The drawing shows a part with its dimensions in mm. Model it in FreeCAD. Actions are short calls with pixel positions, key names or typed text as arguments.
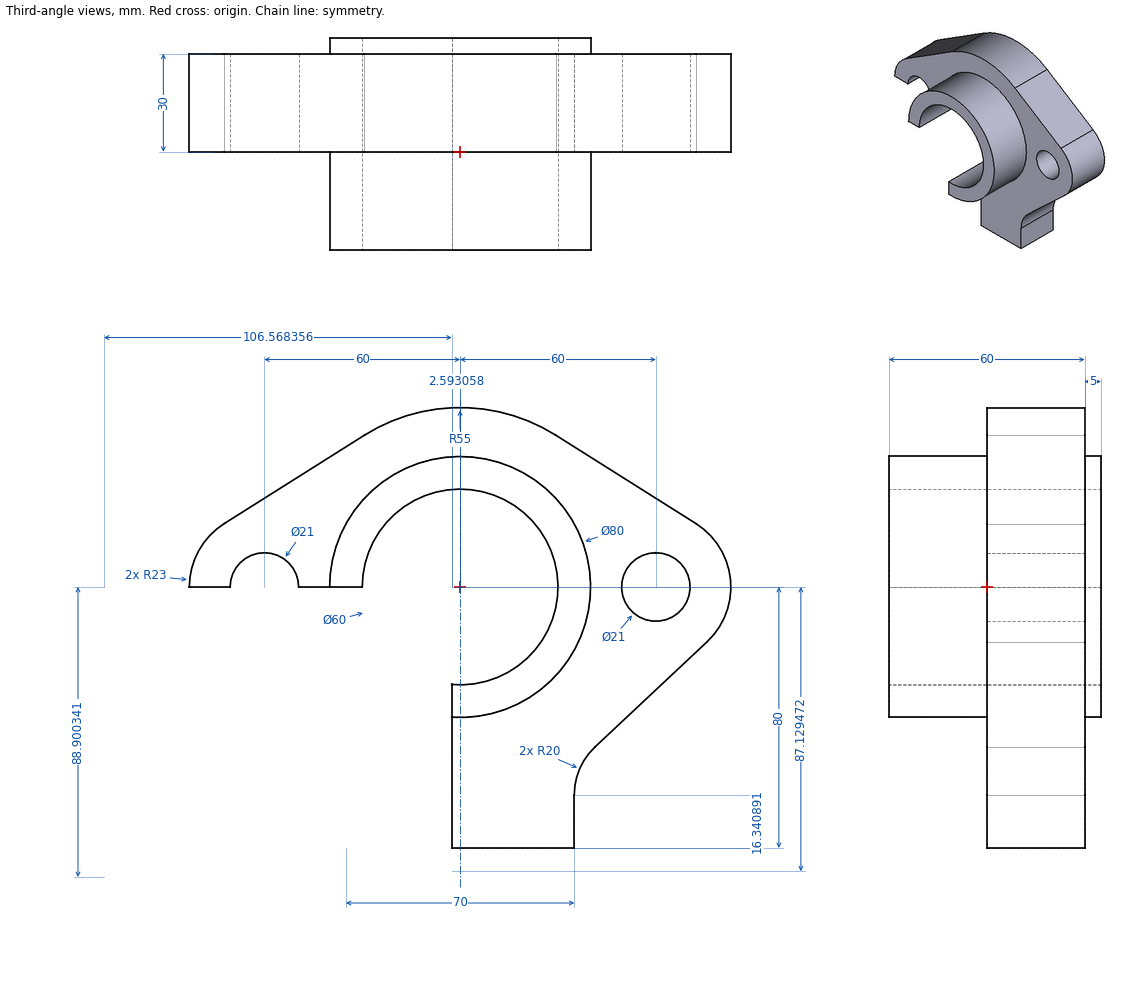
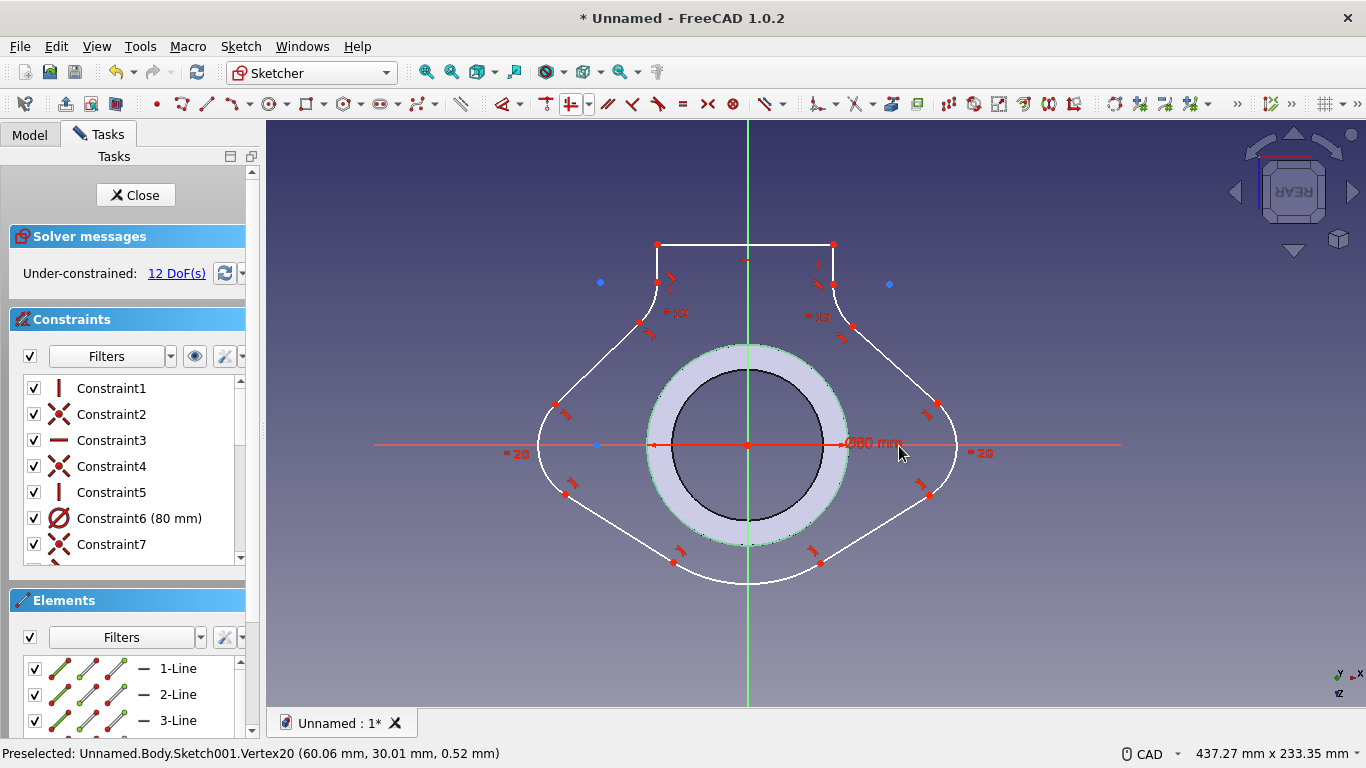
click(424, 445)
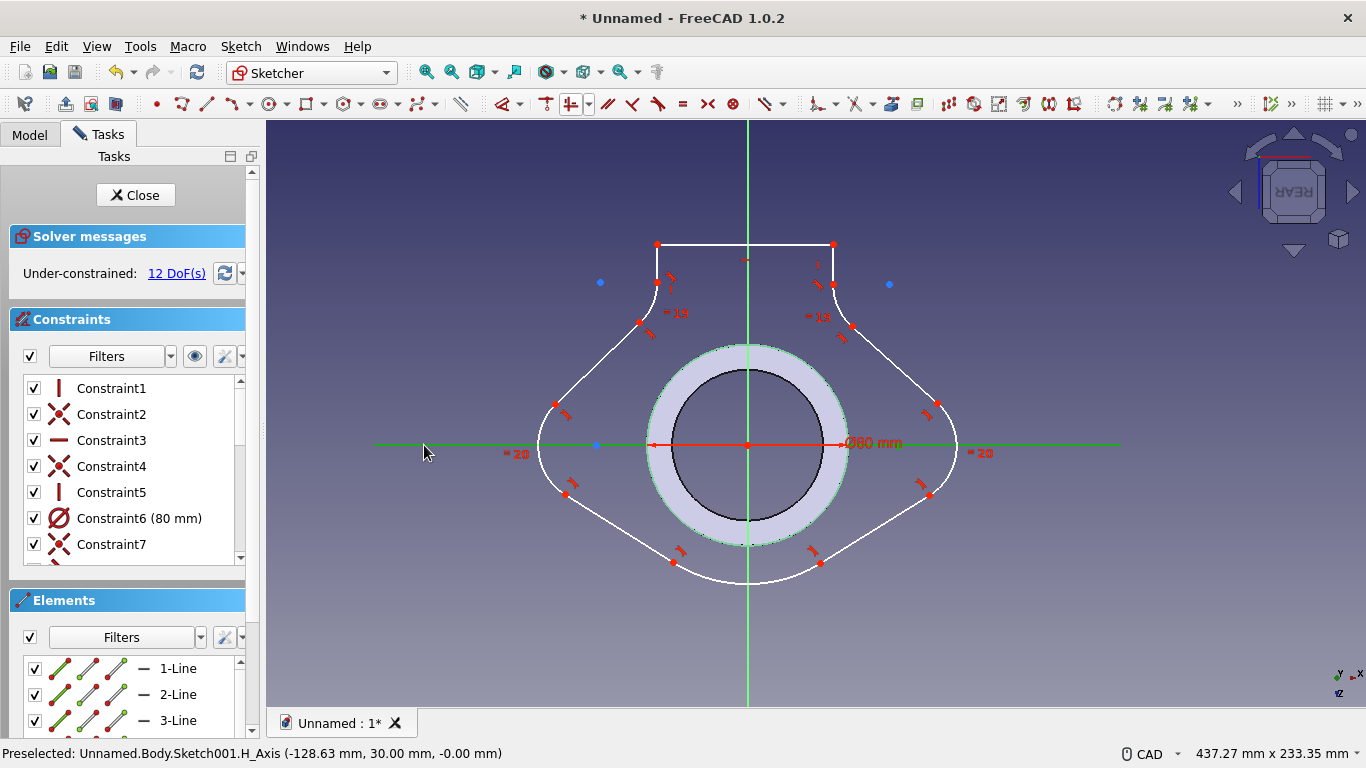
click(546, 104)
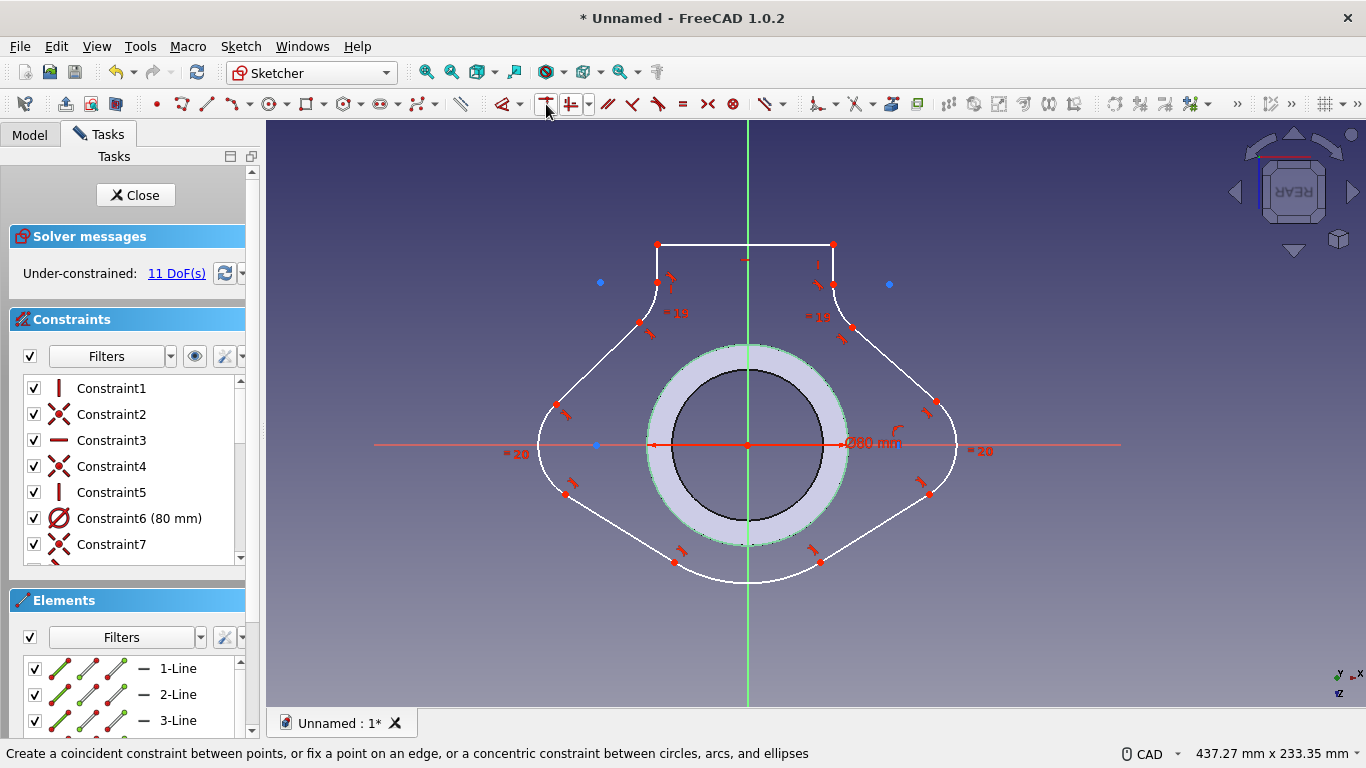
click(596, 446)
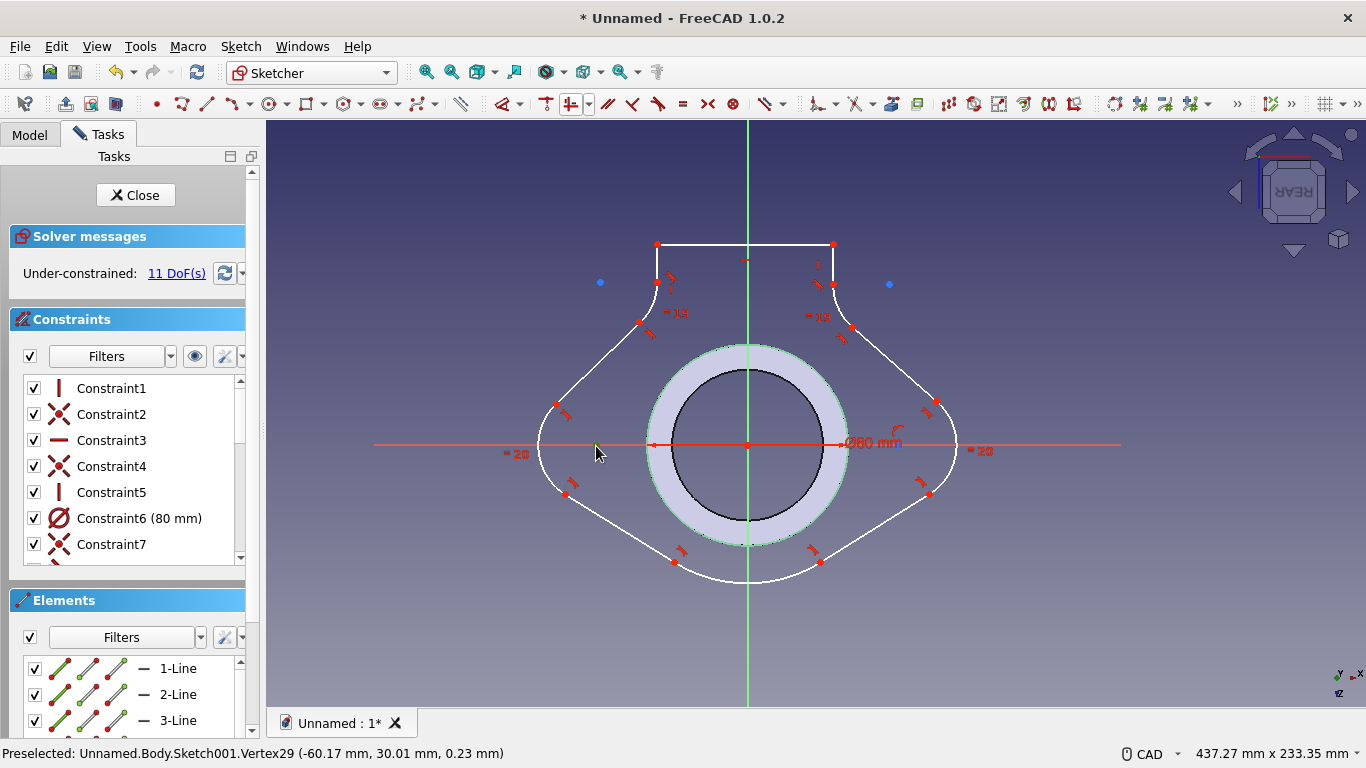
click(424, 445)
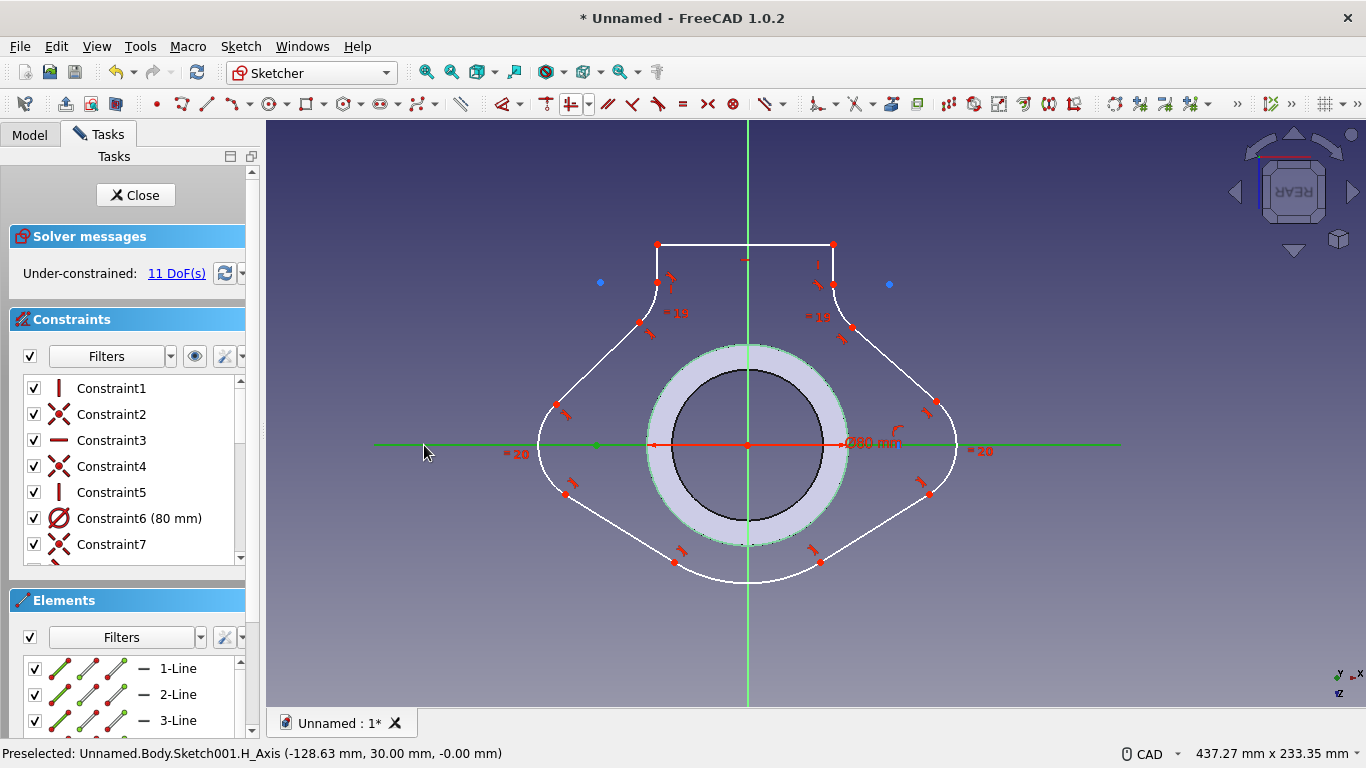
click(546, 104)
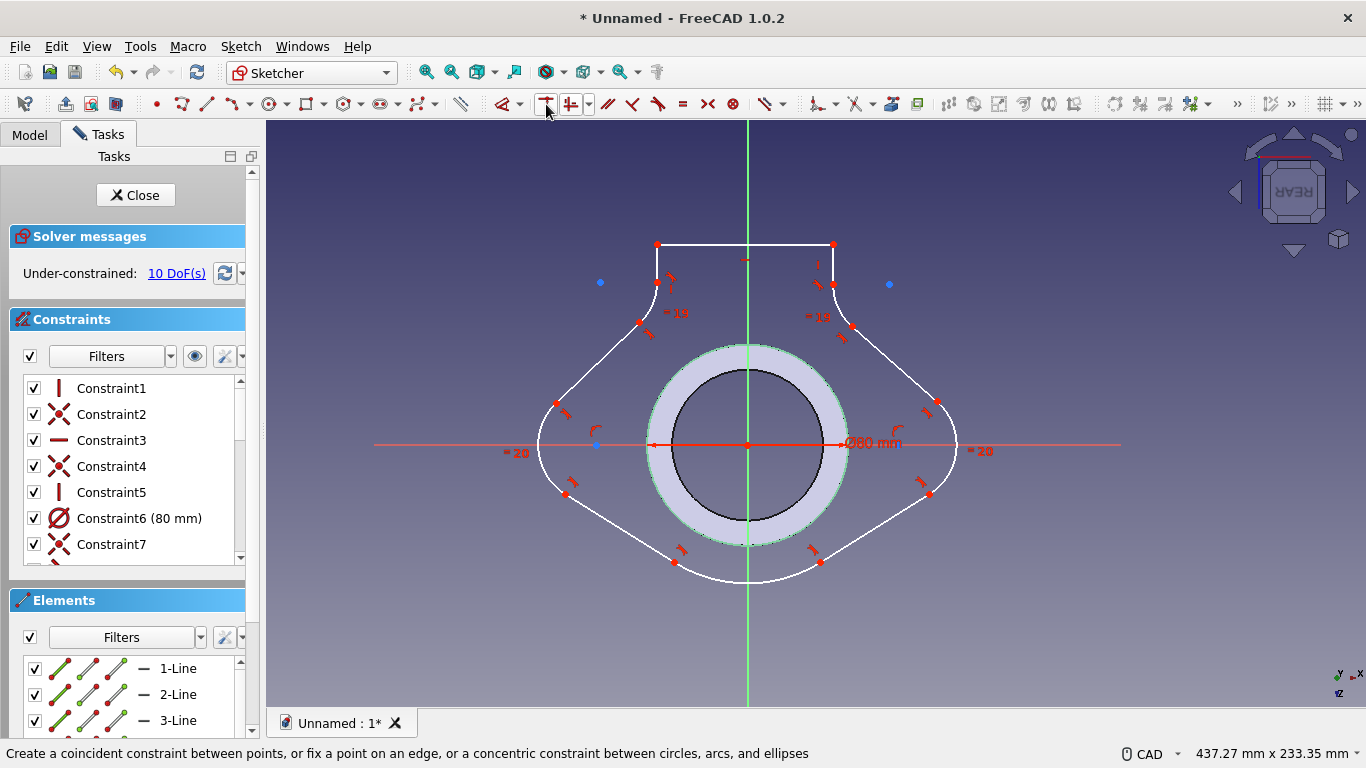
click(890, 285)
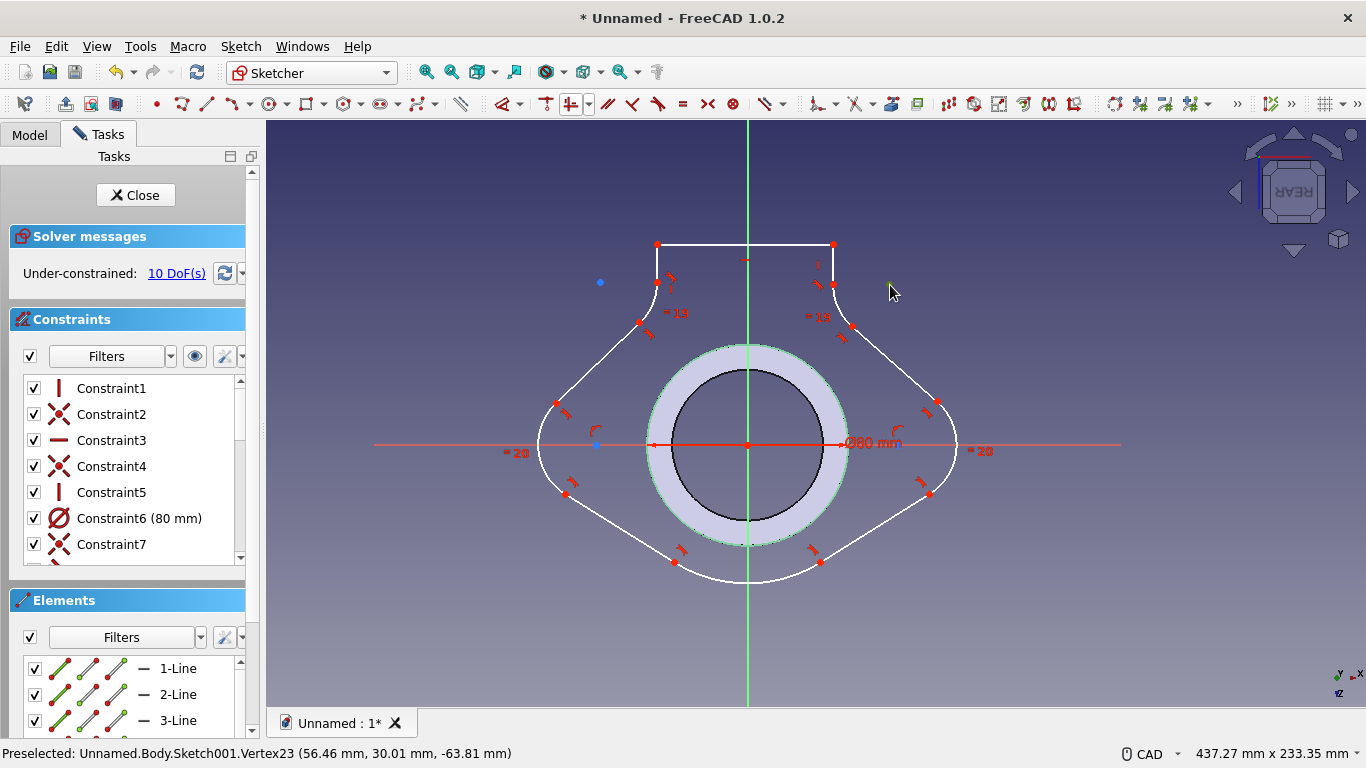
click(601, 282)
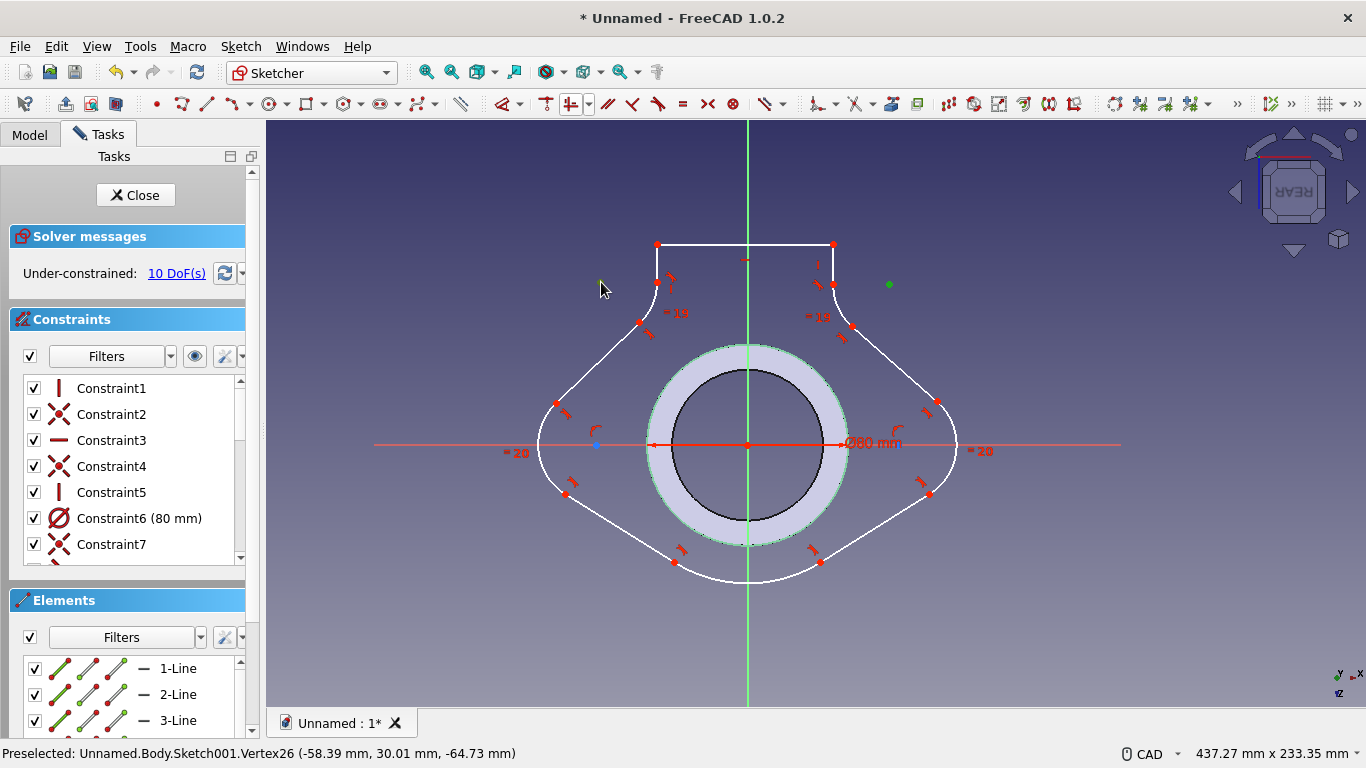
click(748, 641)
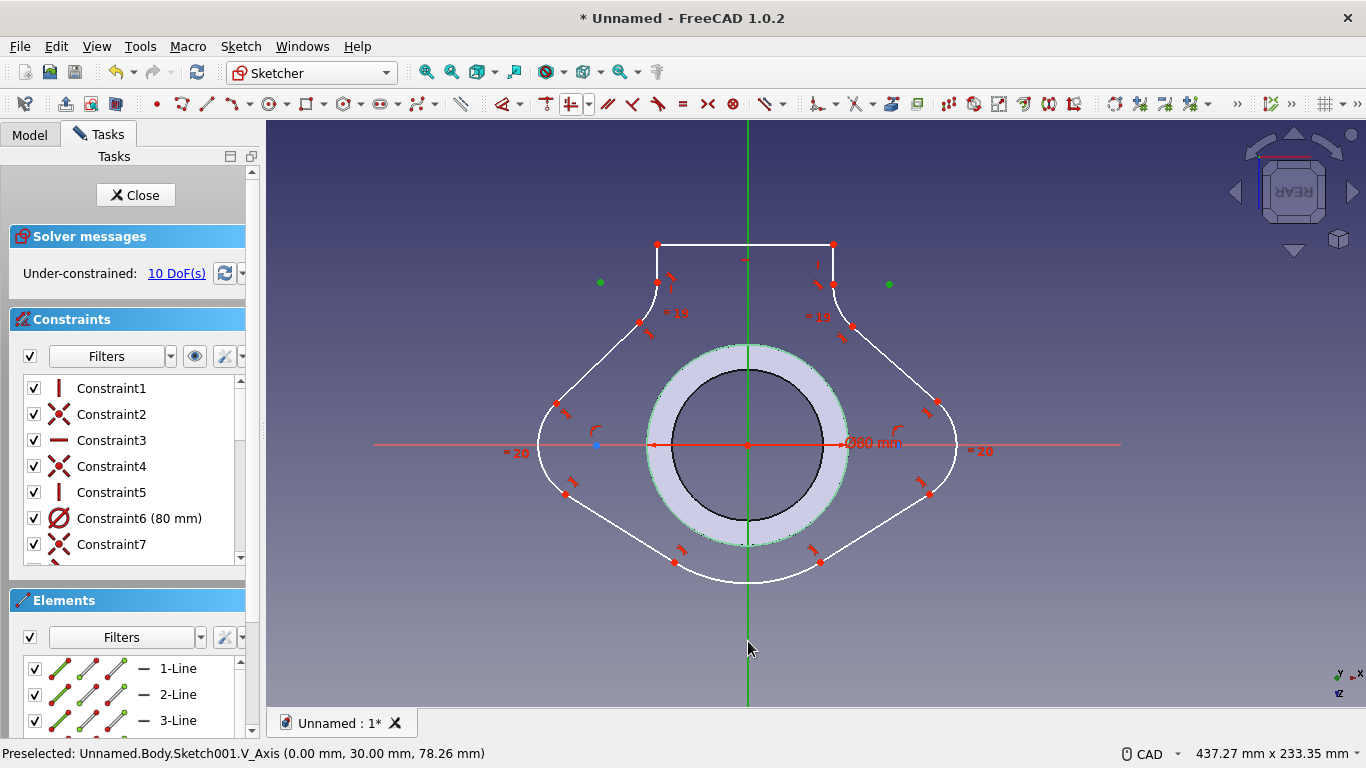
click(708, 104)